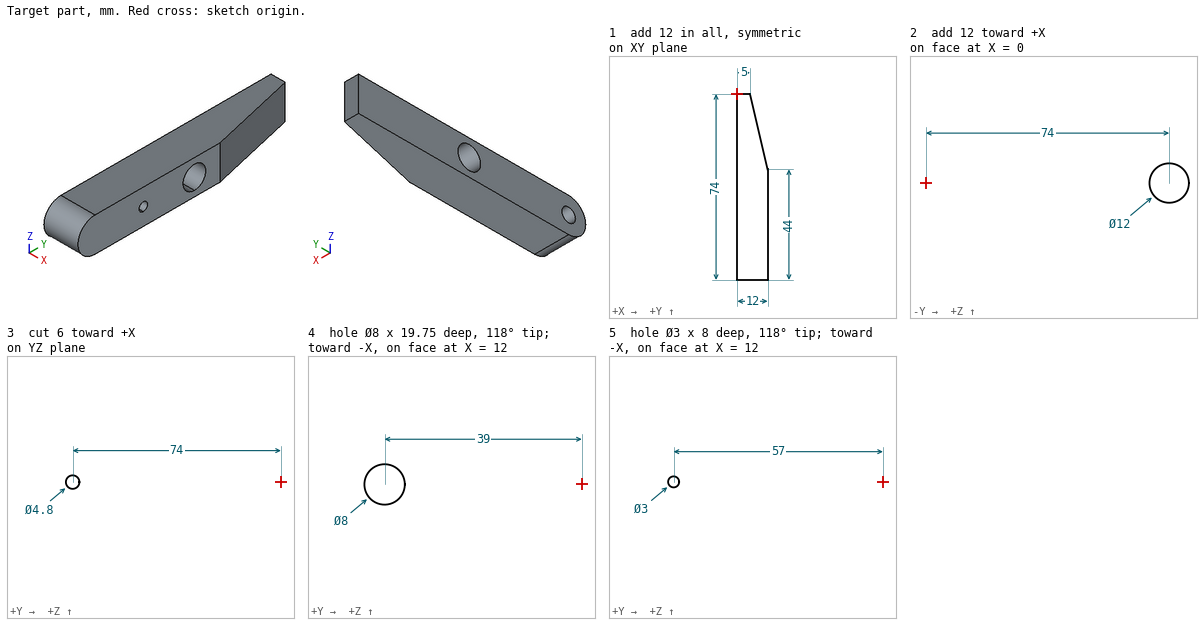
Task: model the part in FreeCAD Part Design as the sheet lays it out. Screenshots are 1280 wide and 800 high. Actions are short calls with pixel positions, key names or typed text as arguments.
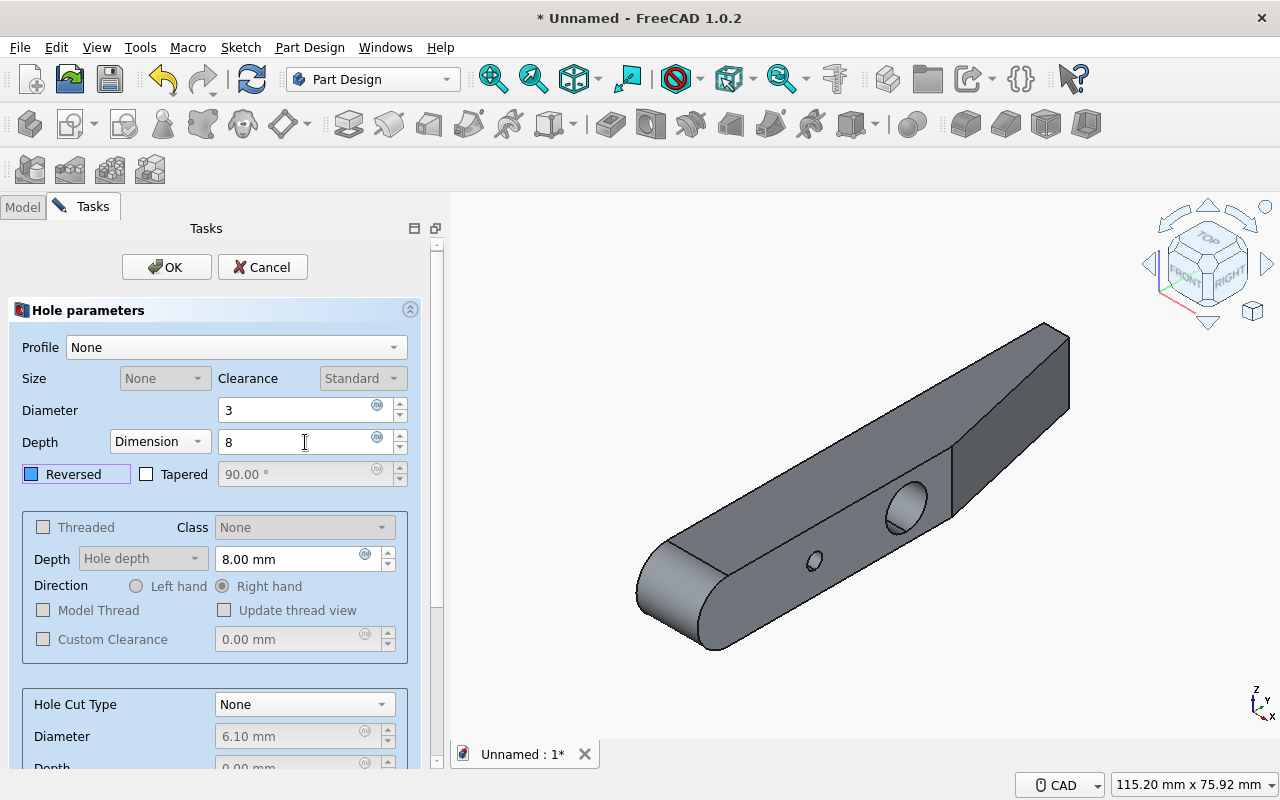
click(167, 267)